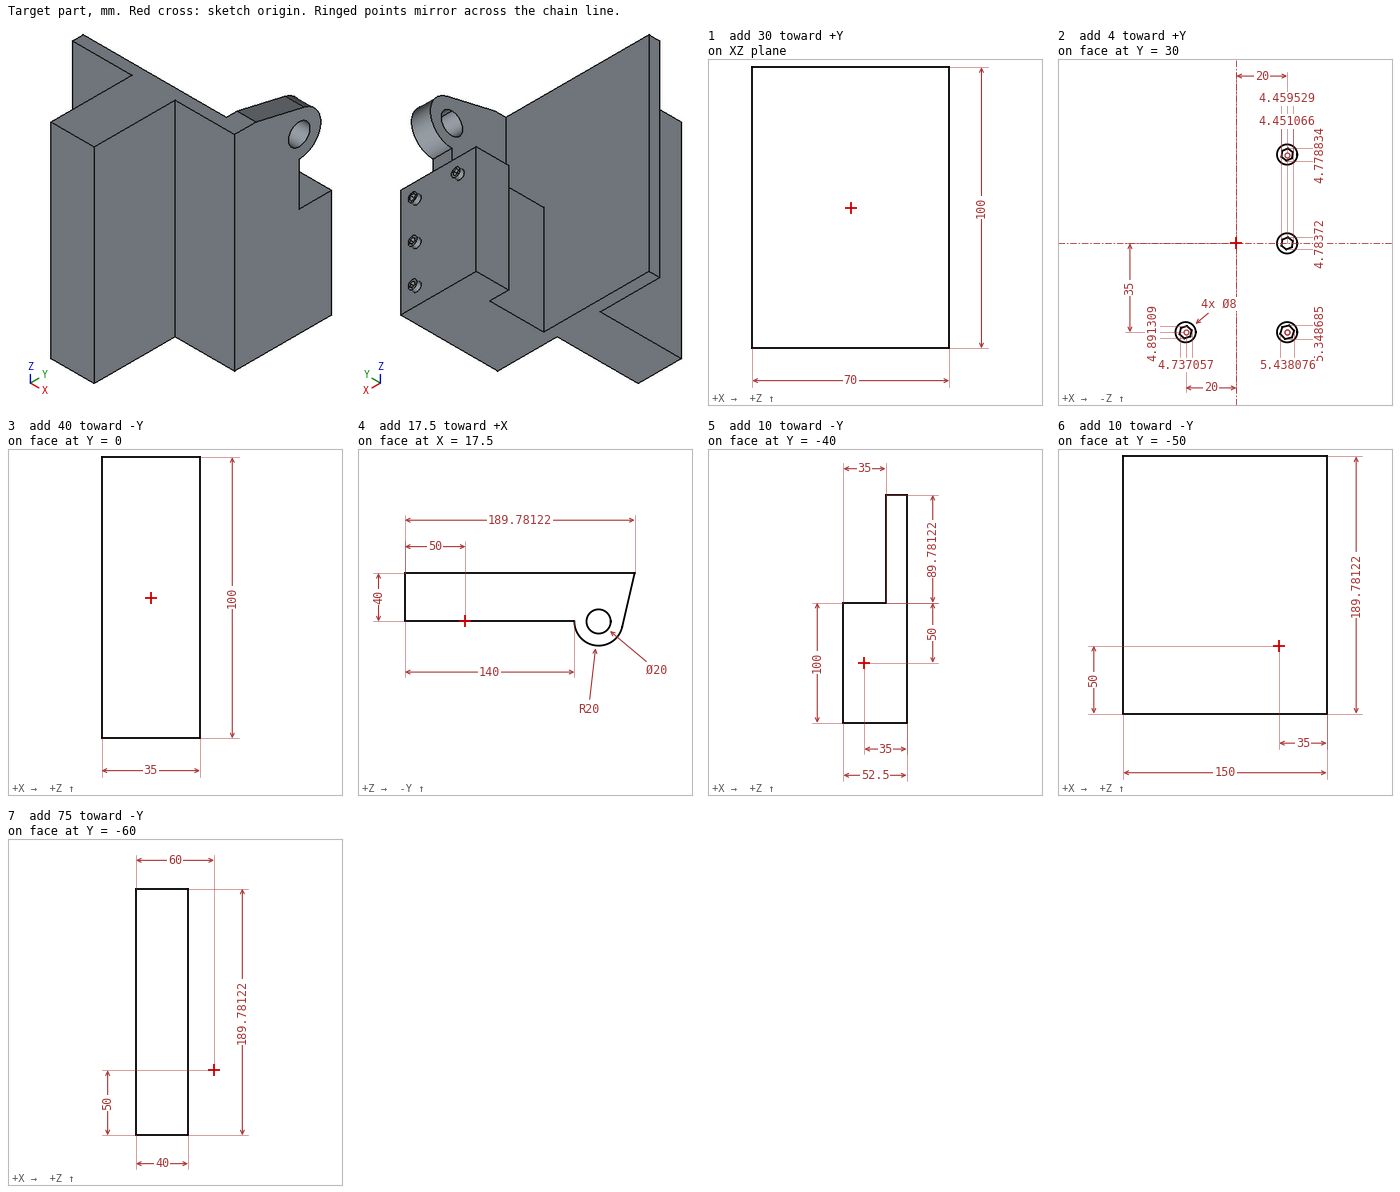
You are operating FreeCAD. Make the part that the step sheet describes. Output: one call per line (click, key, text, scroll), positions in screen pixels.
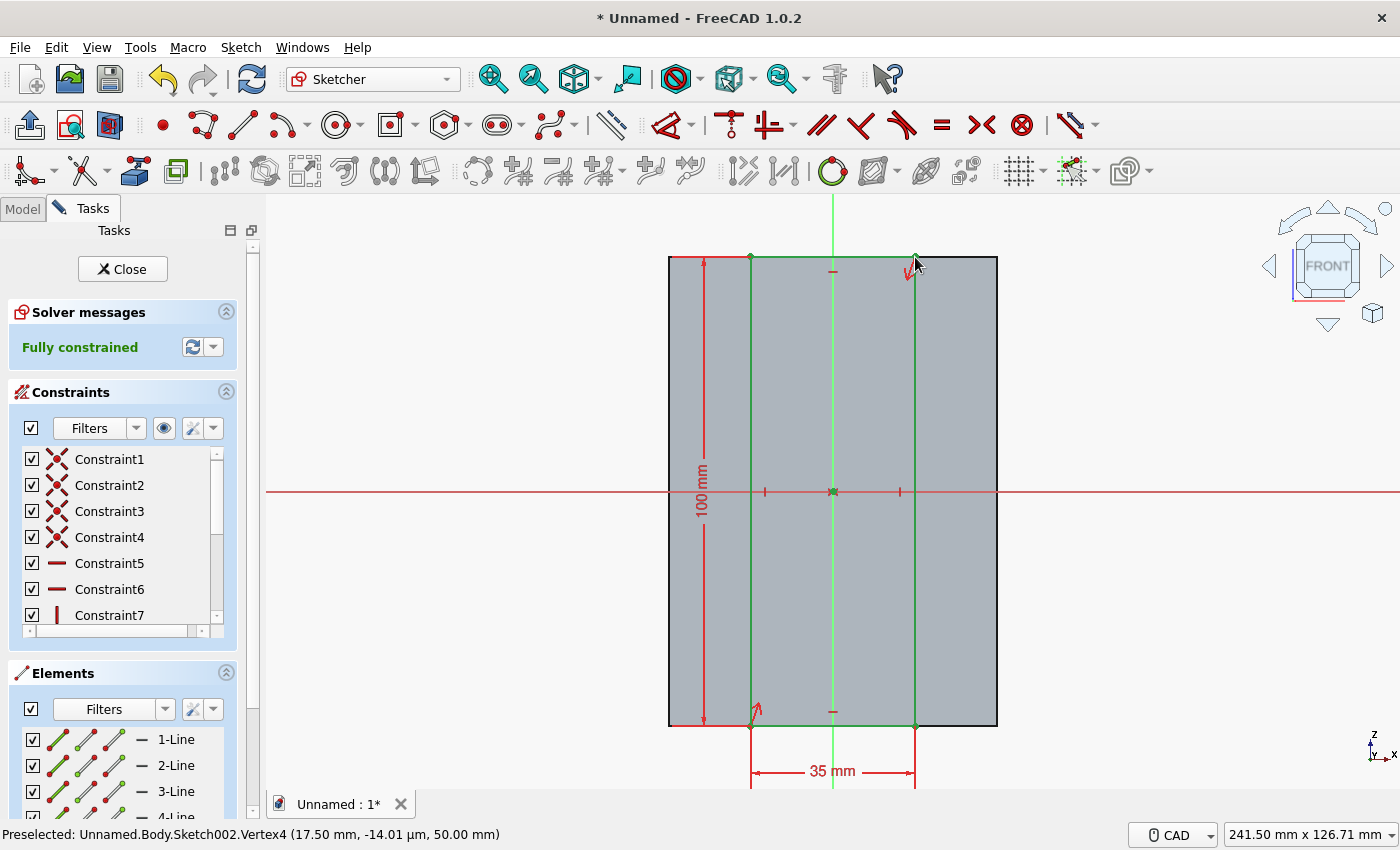
click(123, 269)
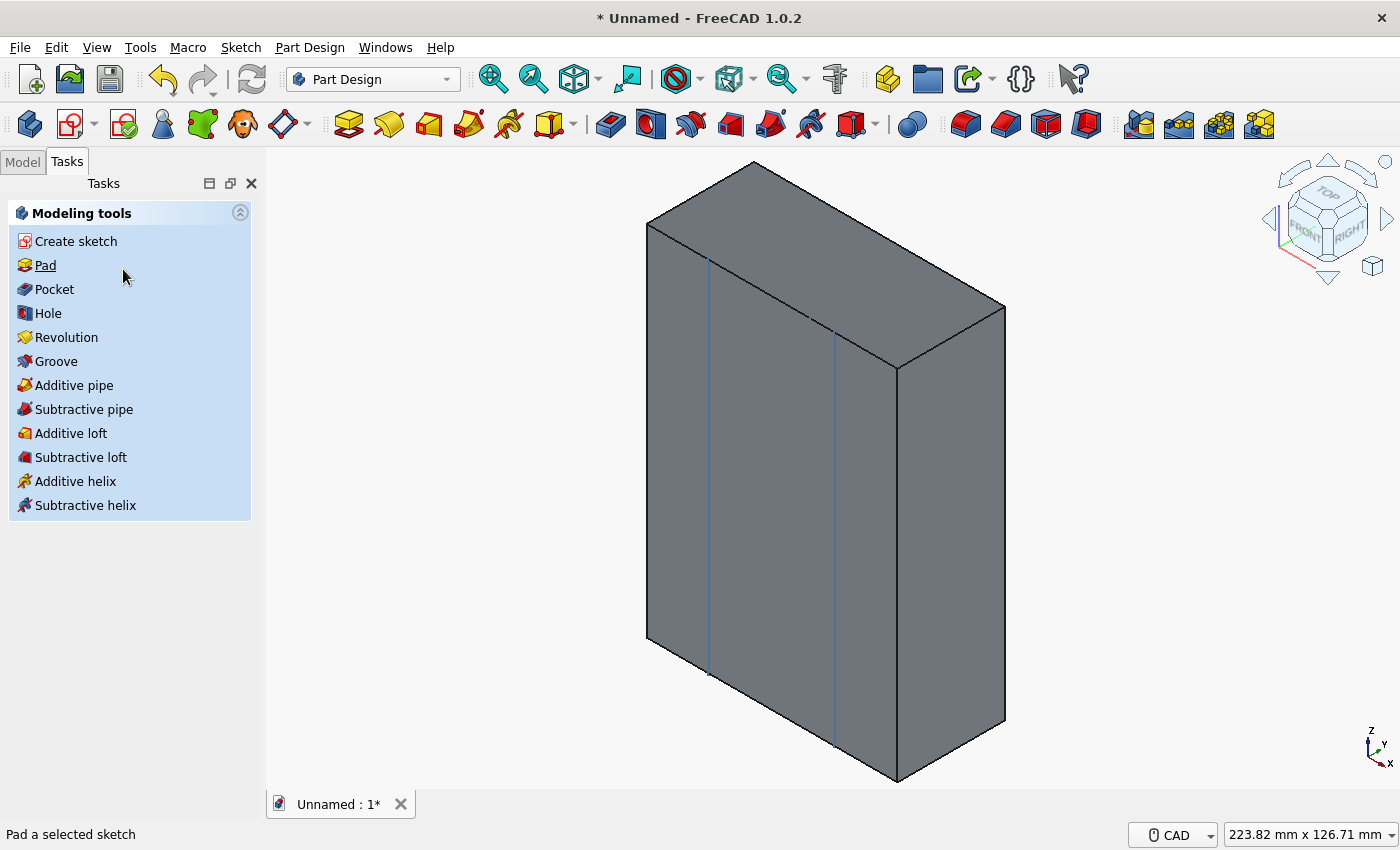
click(350, 124)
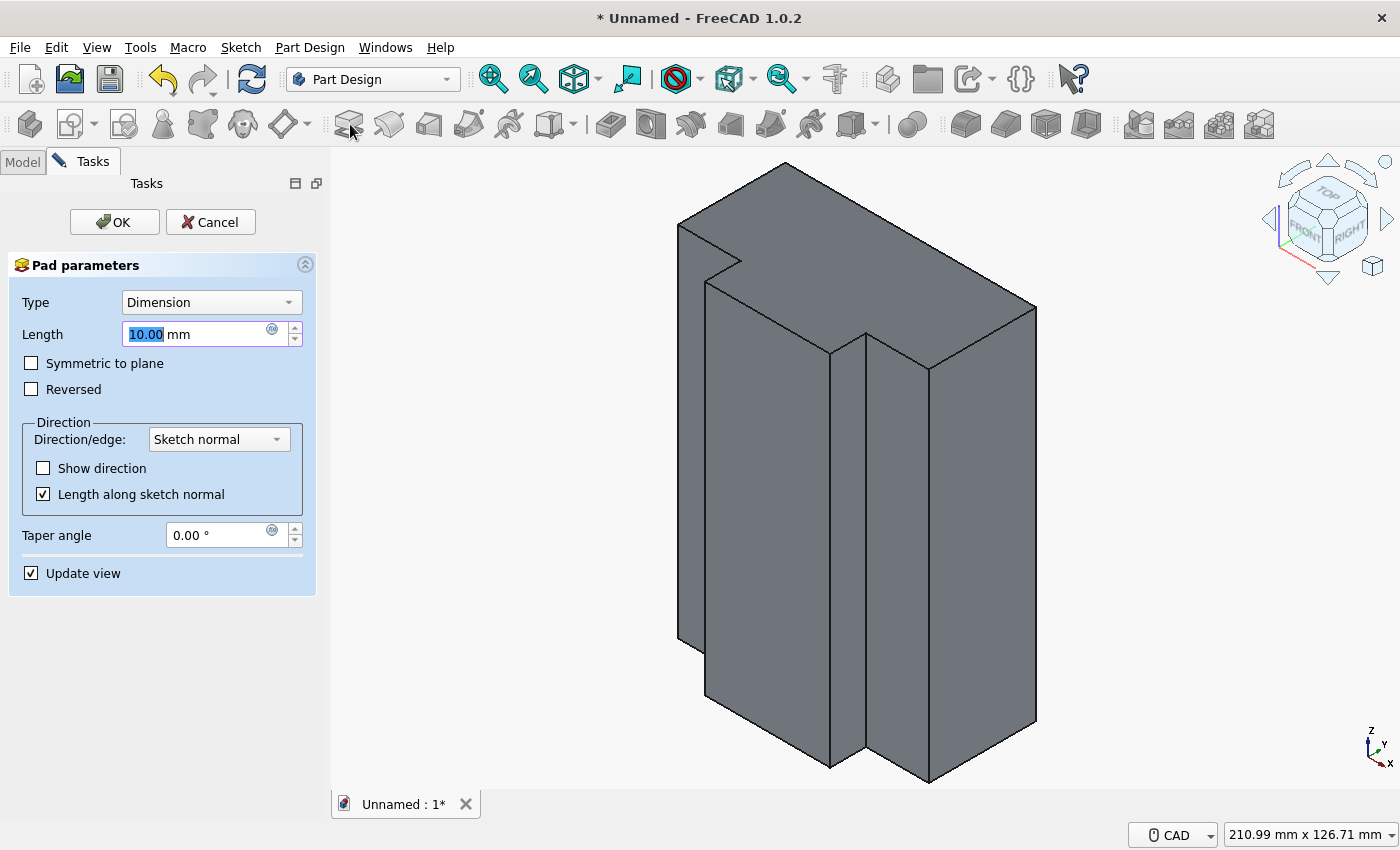
text(40)
key(Tab)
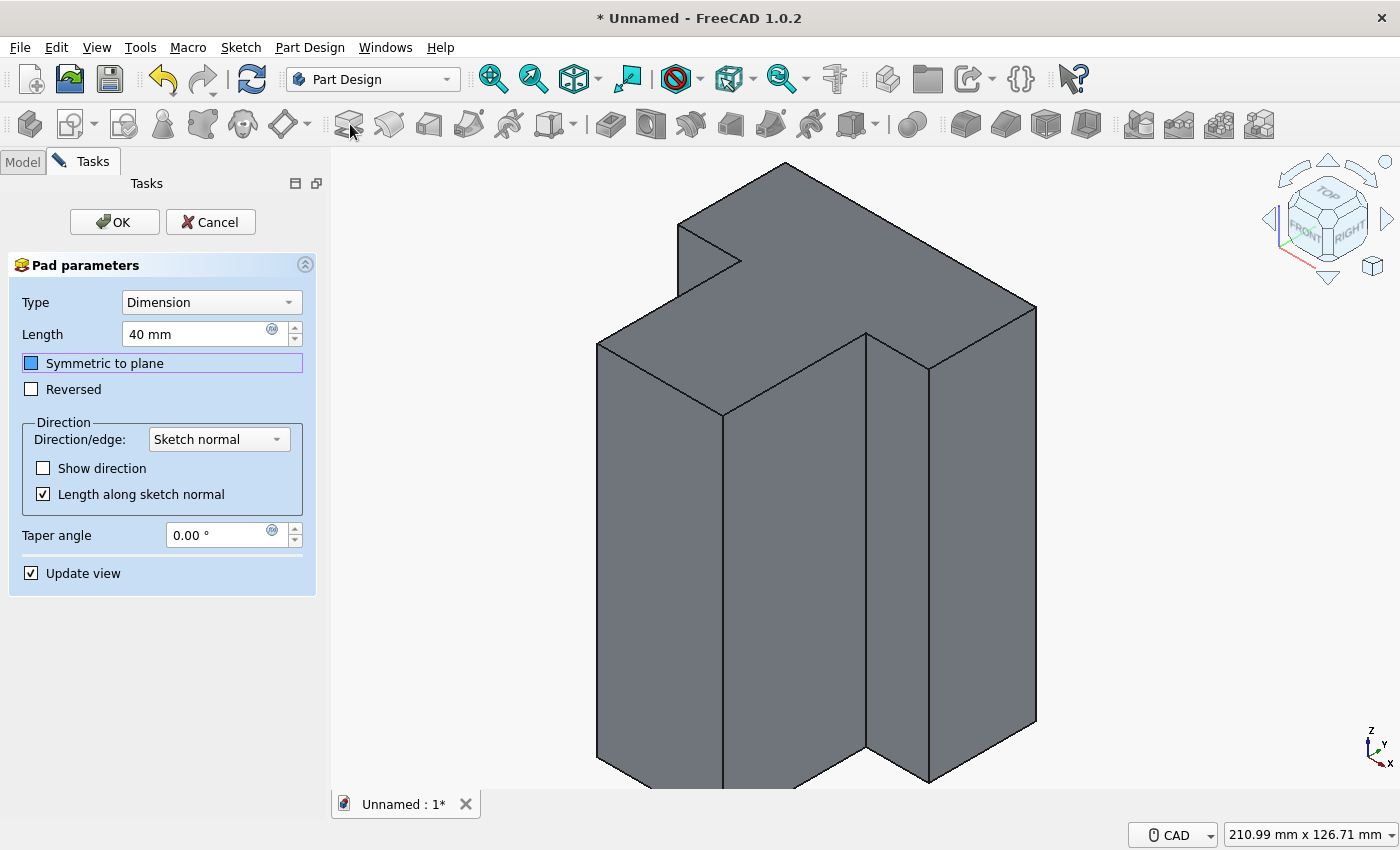
click(115, 222)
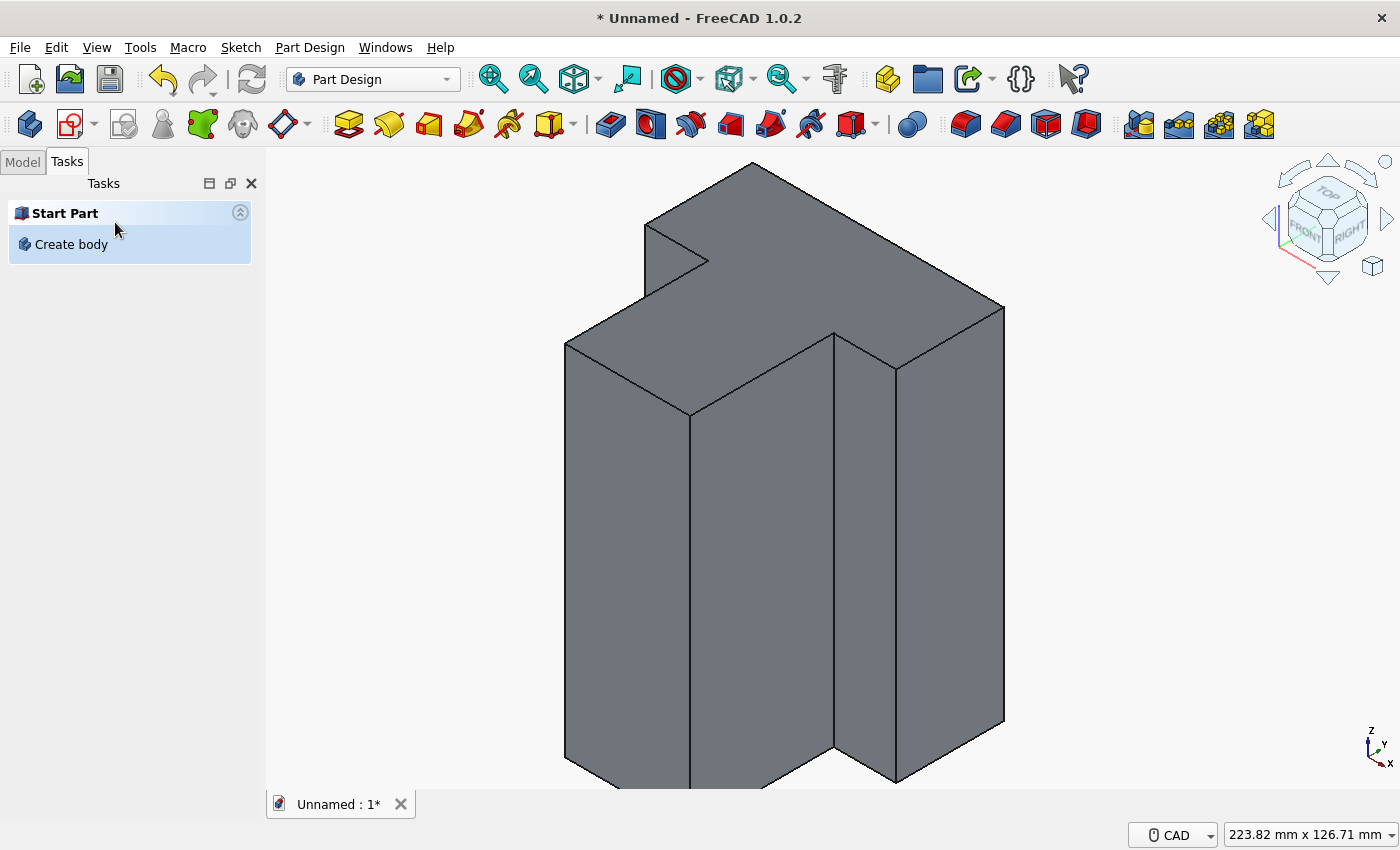
click(494, 80)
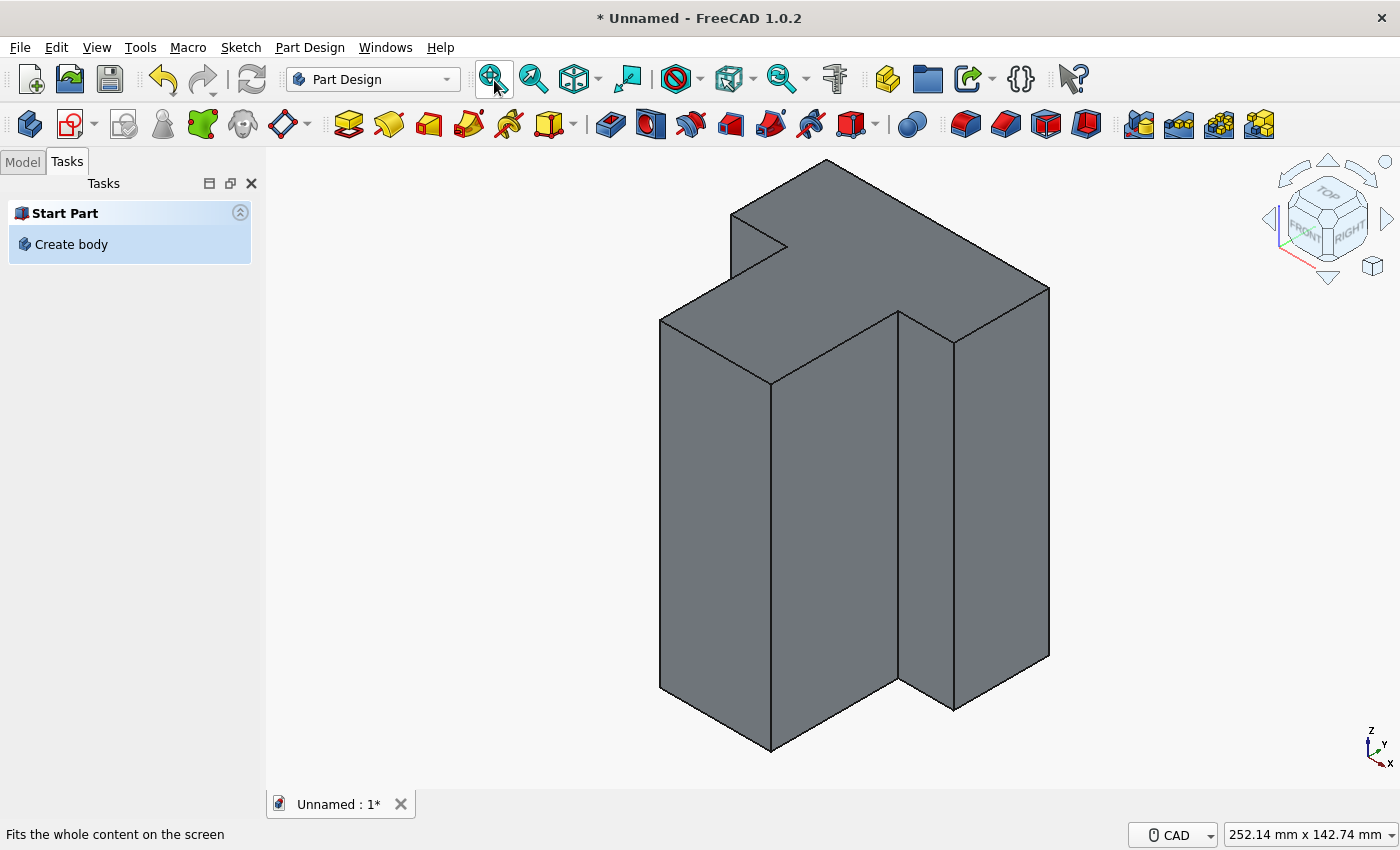
click(835, 425)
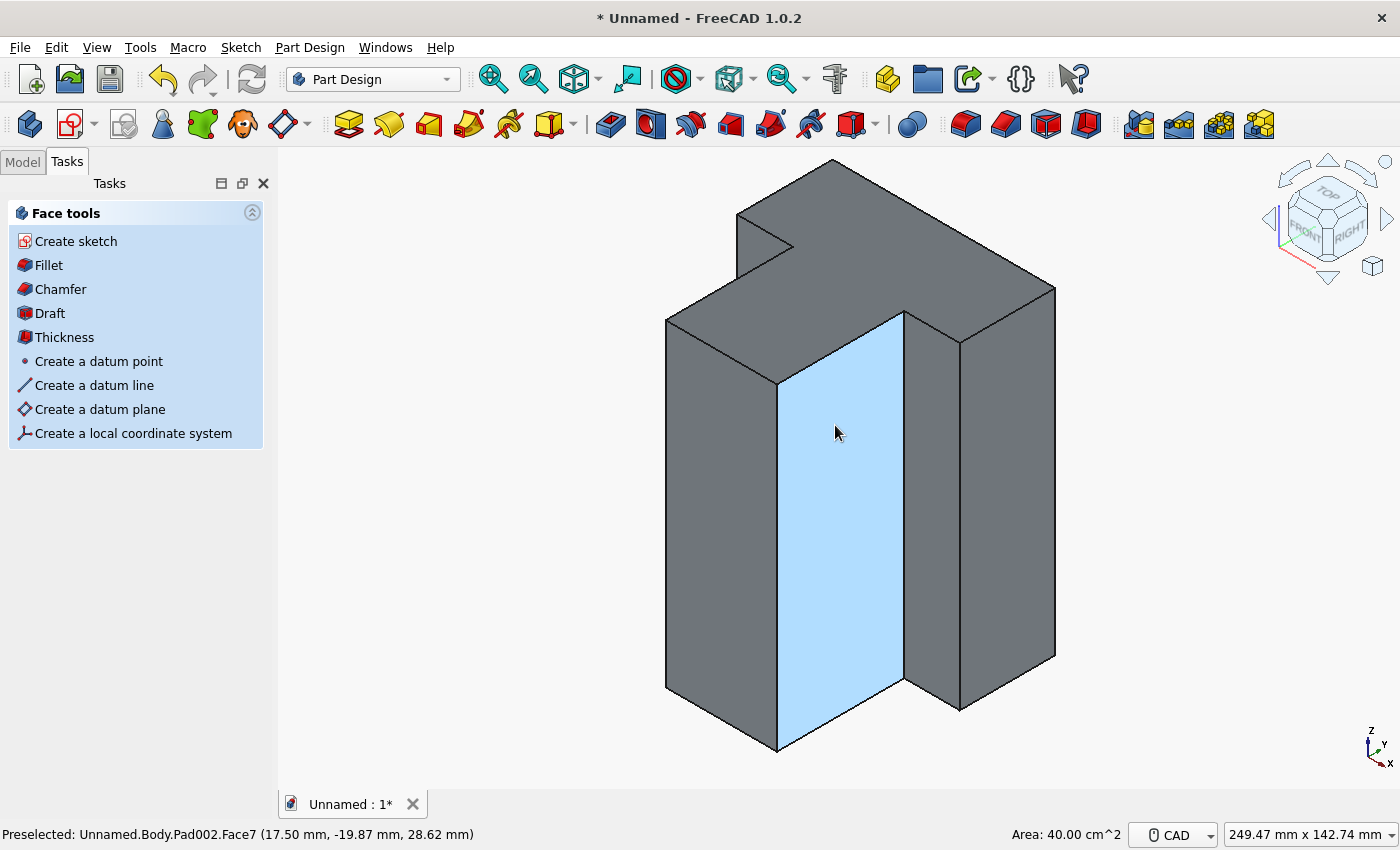
click(70, 124)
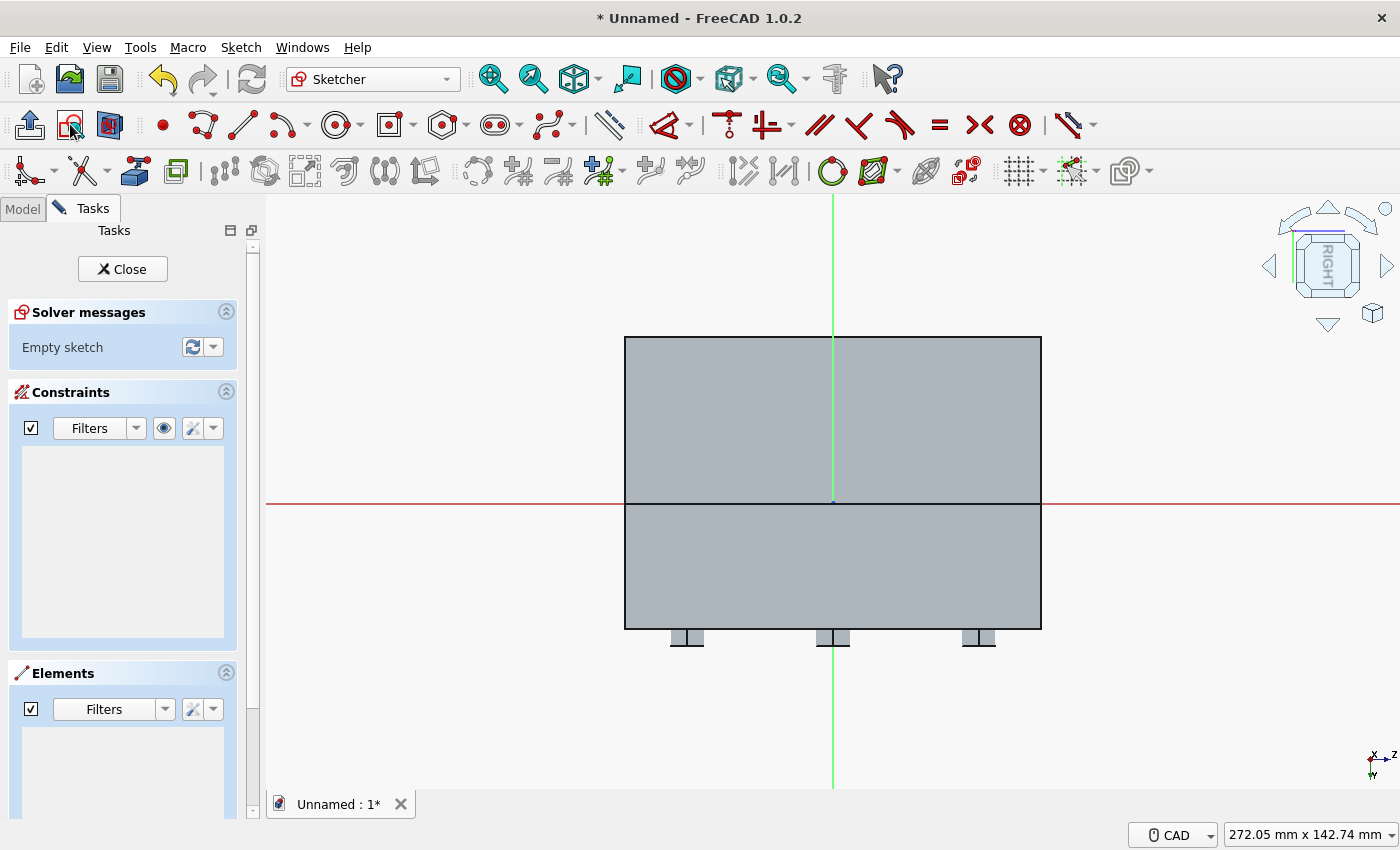
click(110, 126)